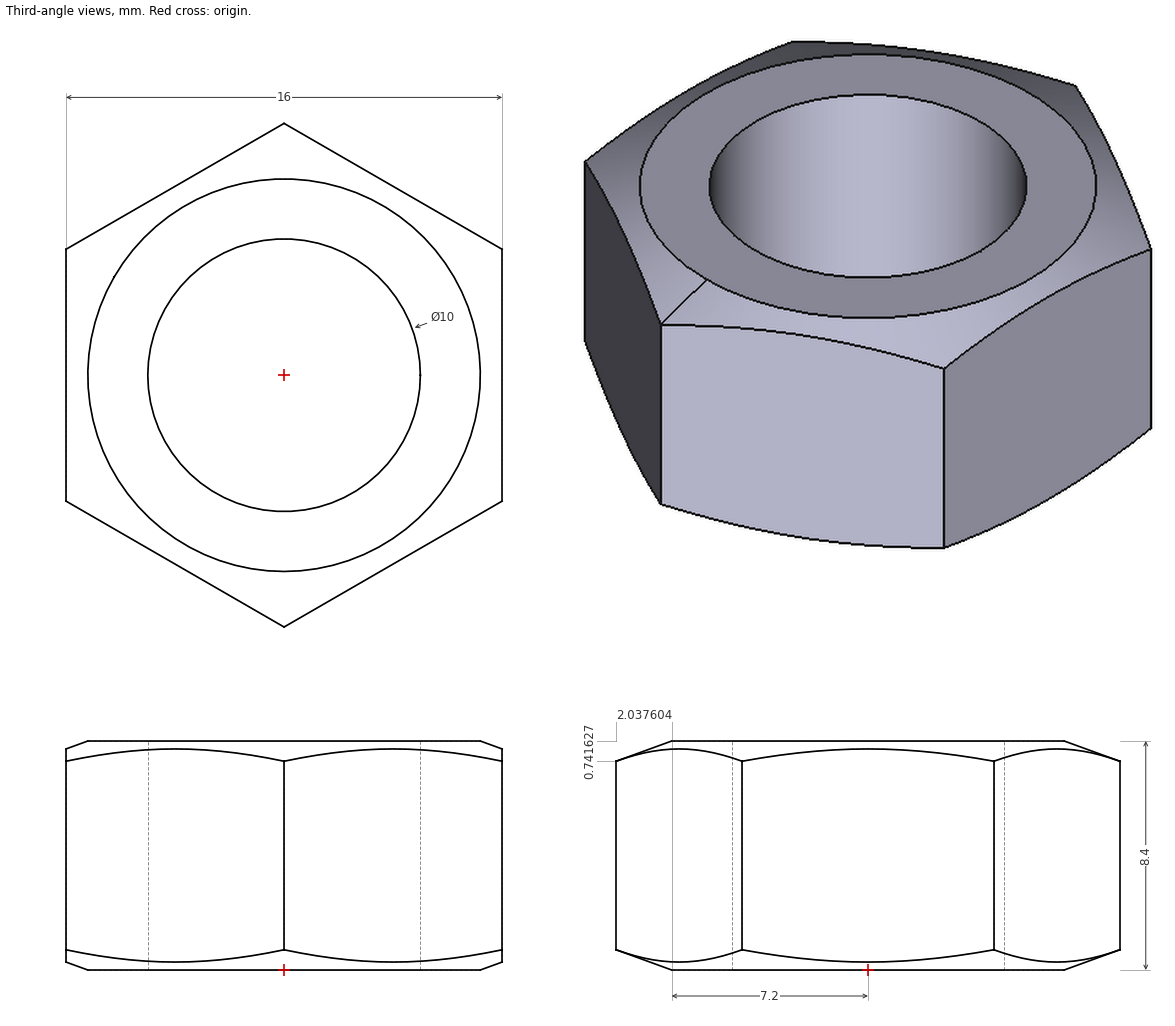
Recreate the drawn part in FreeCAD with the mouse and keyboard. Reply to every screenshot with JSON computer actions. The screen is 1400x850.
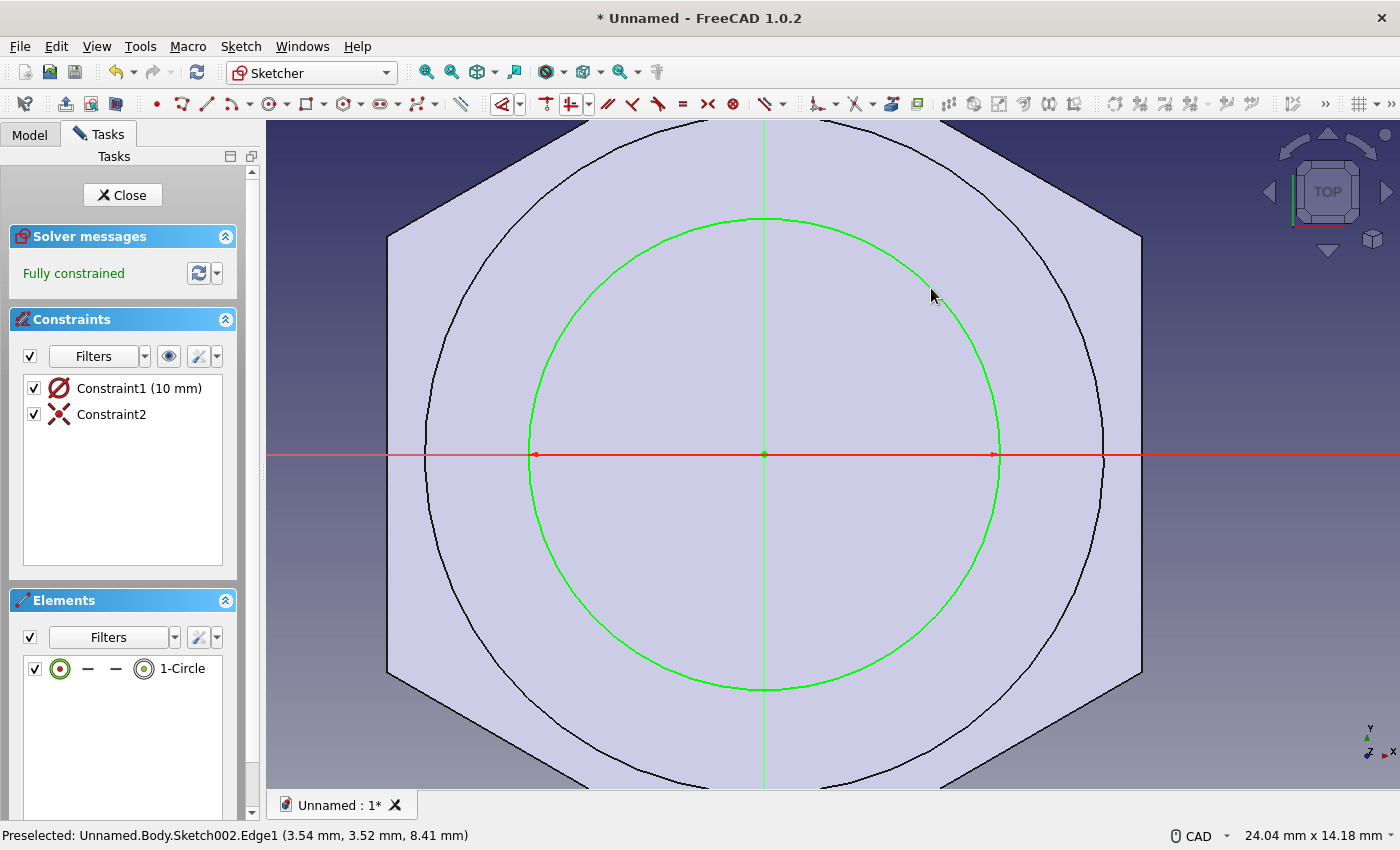
{"action": "left_click", "coordinate": [123, 195]}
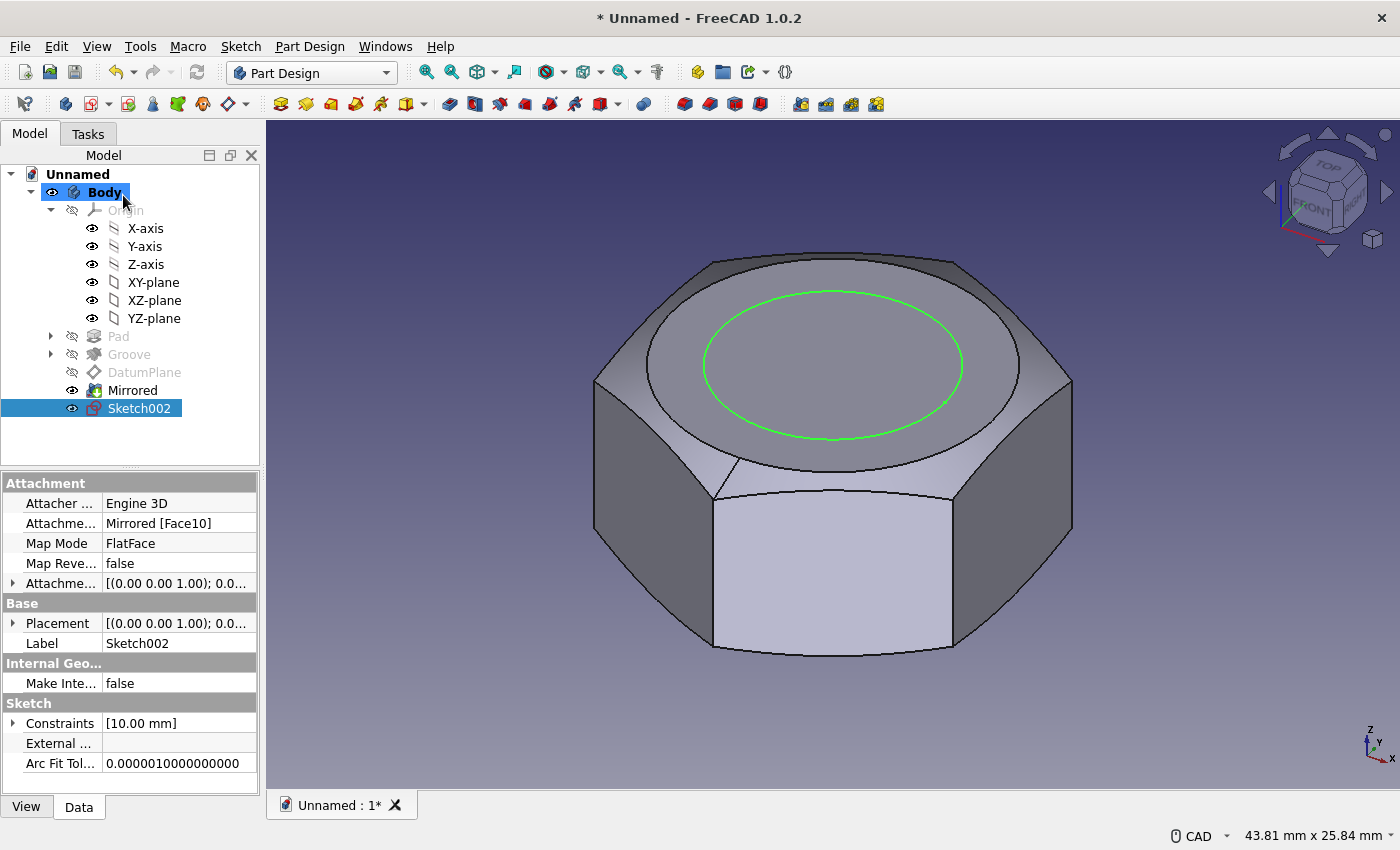
{"action": "left_click", "coordinate": [450, 104]}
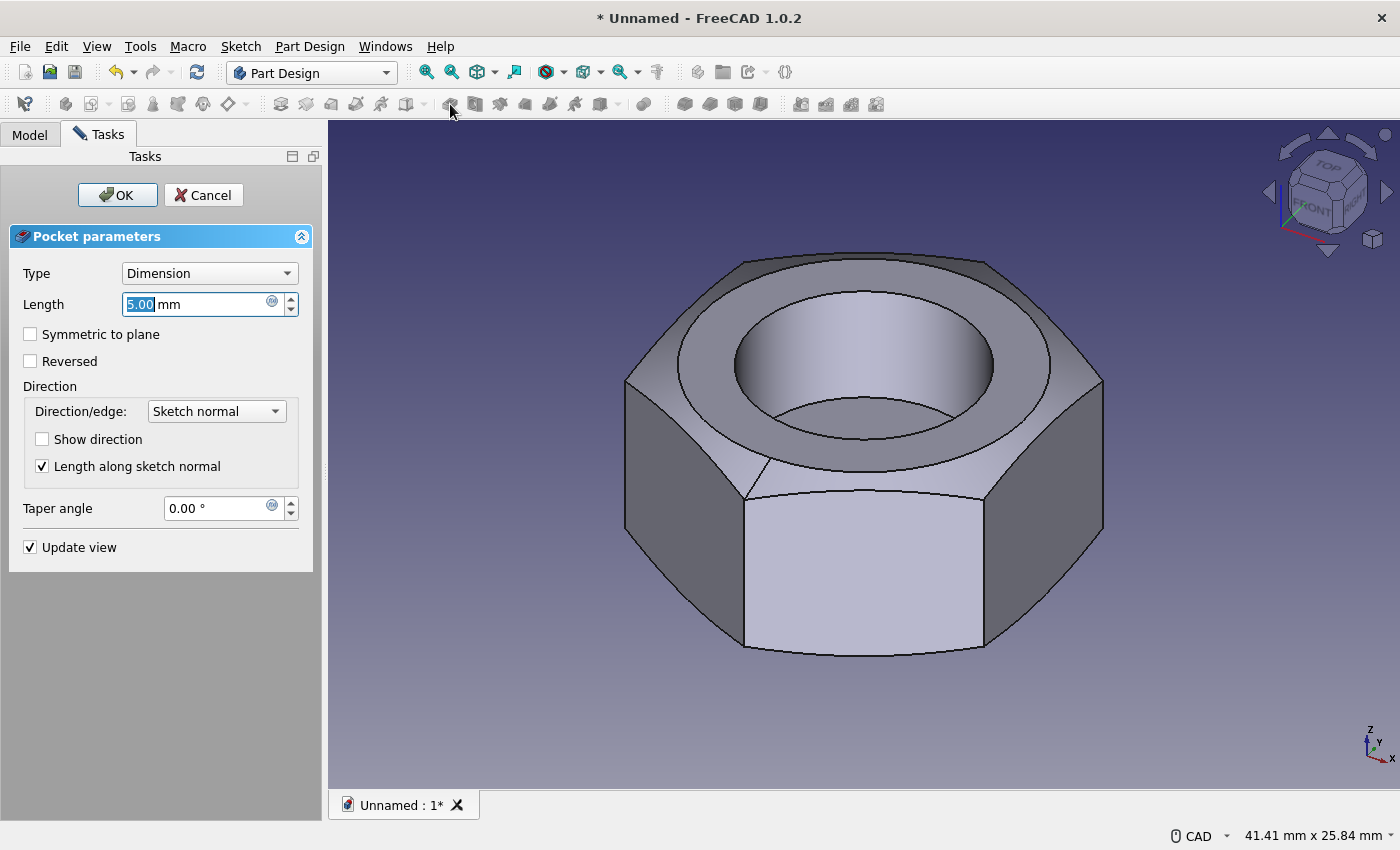
{"action": "left_click", "coordinate": [210, 274]}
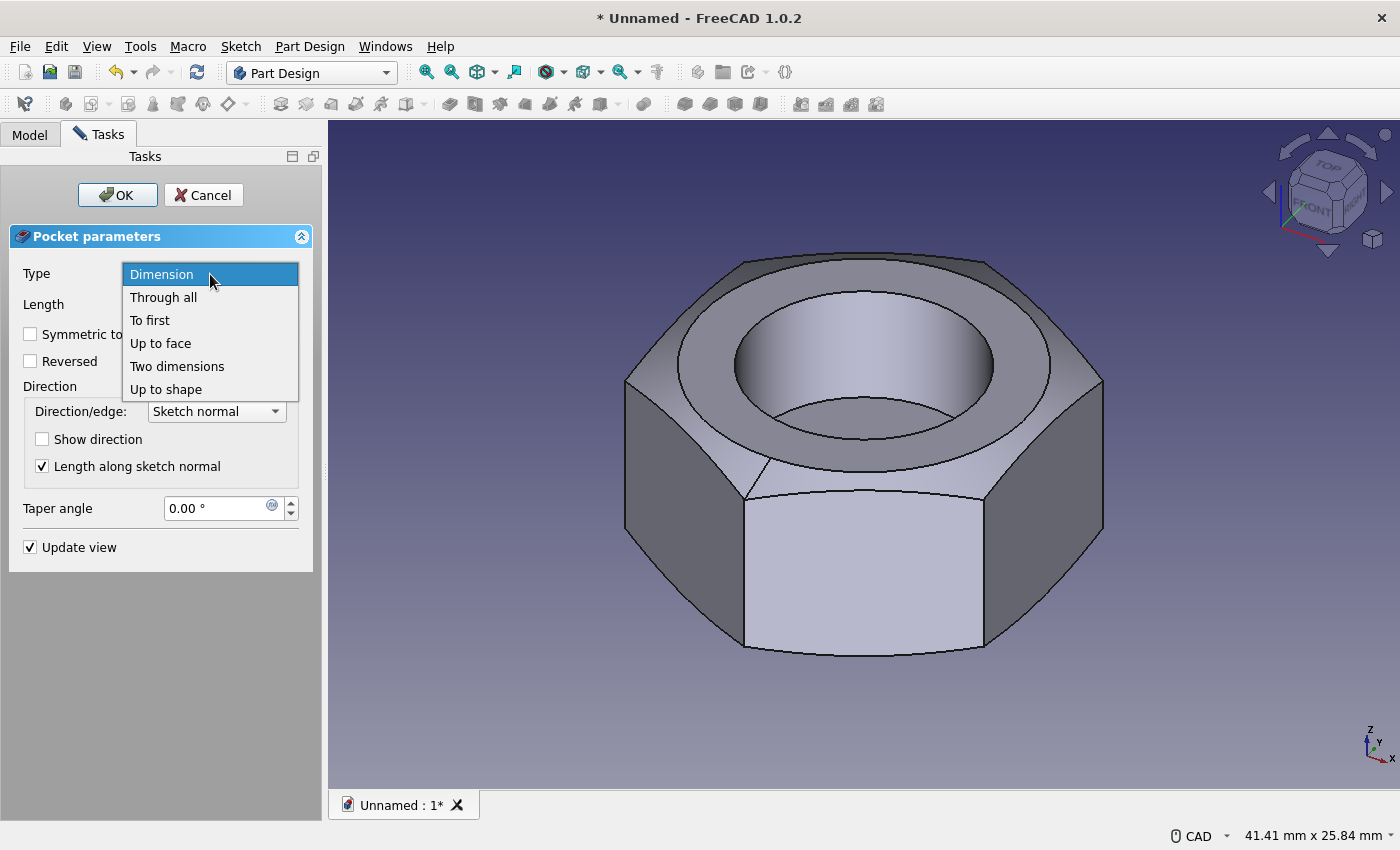
{"action": "left_click", "coordinate": [208, 298]}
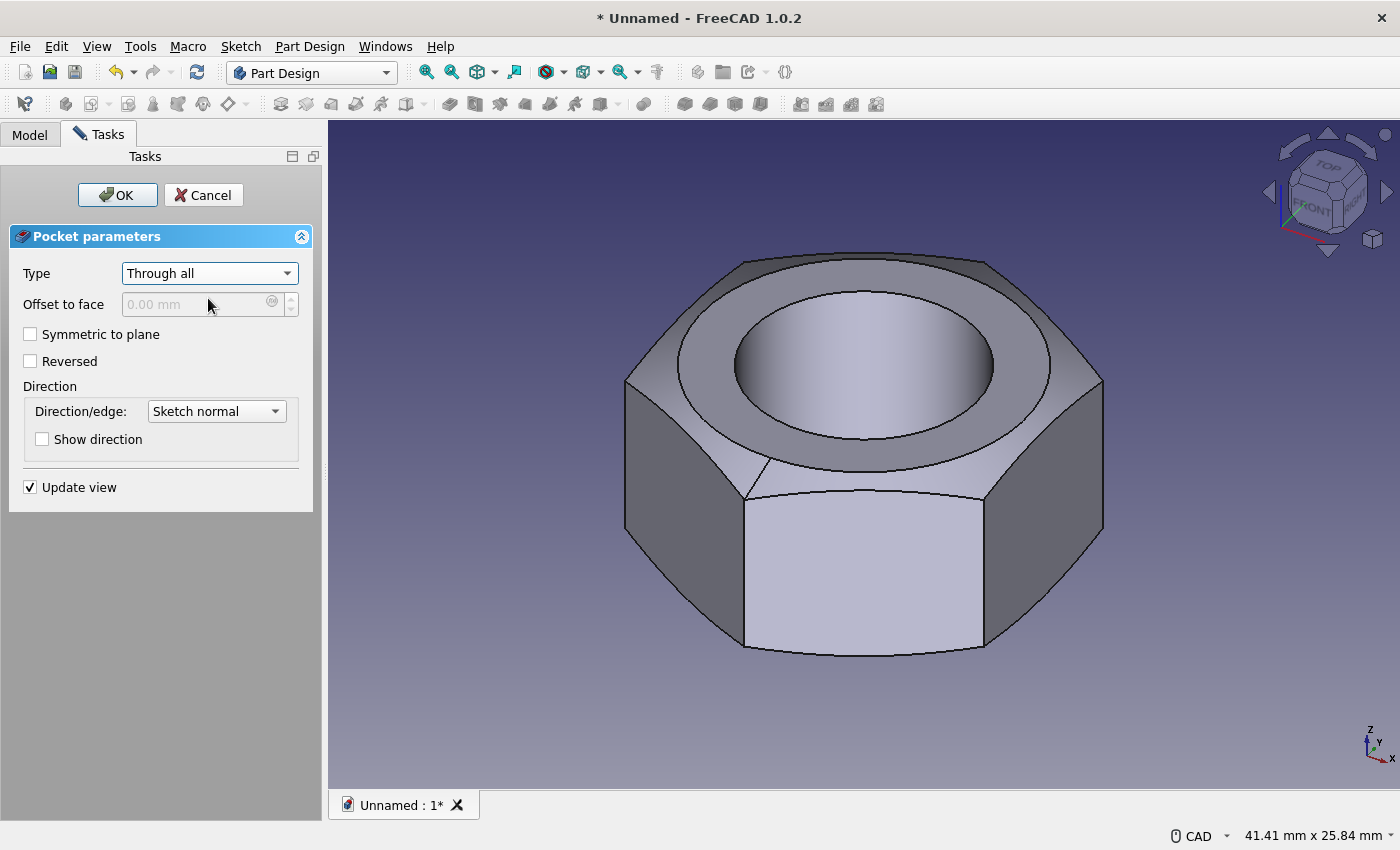
{"action": "left_click", "coordinate": [118, 195]}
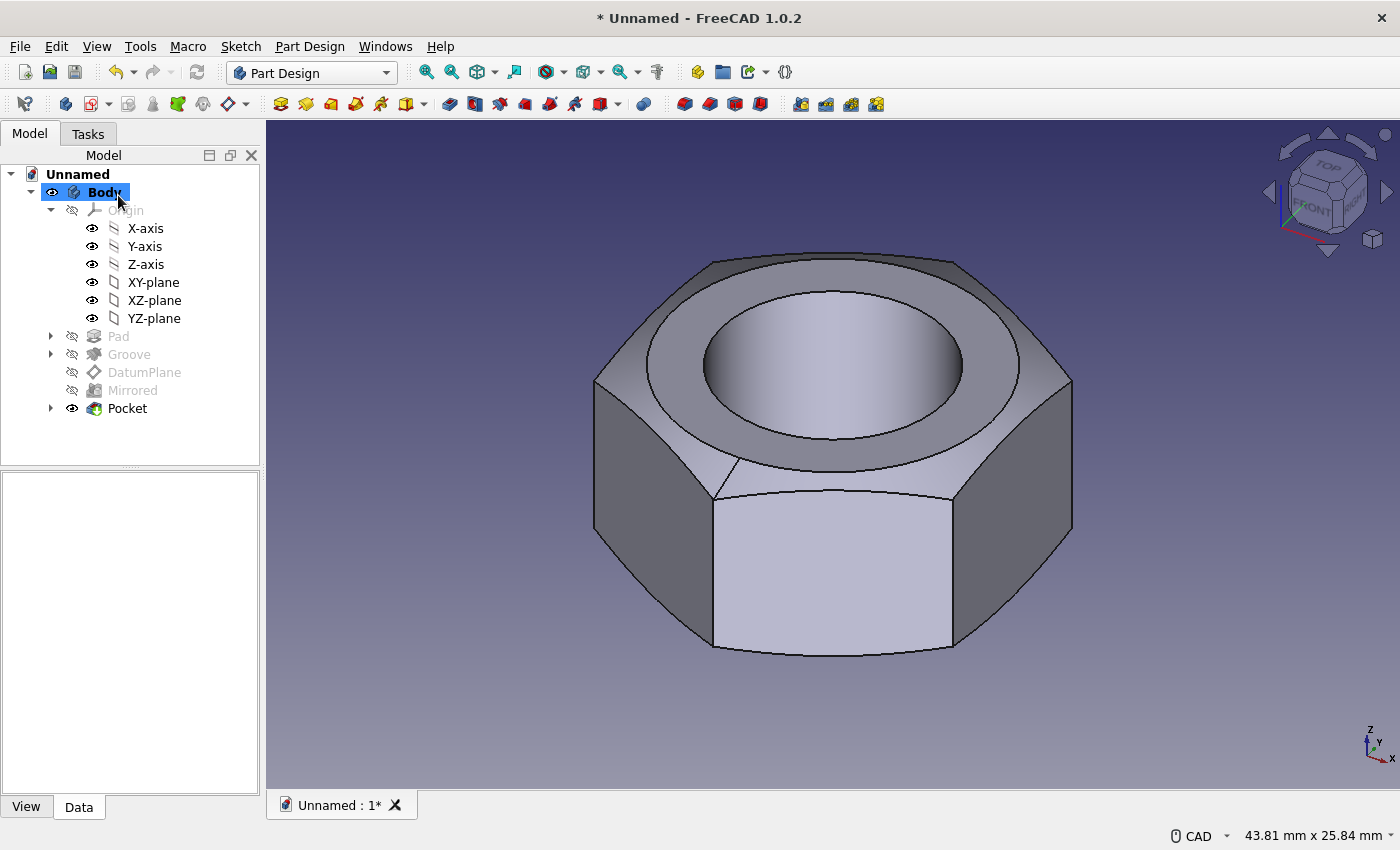
{"action": "key", "text": "0"}